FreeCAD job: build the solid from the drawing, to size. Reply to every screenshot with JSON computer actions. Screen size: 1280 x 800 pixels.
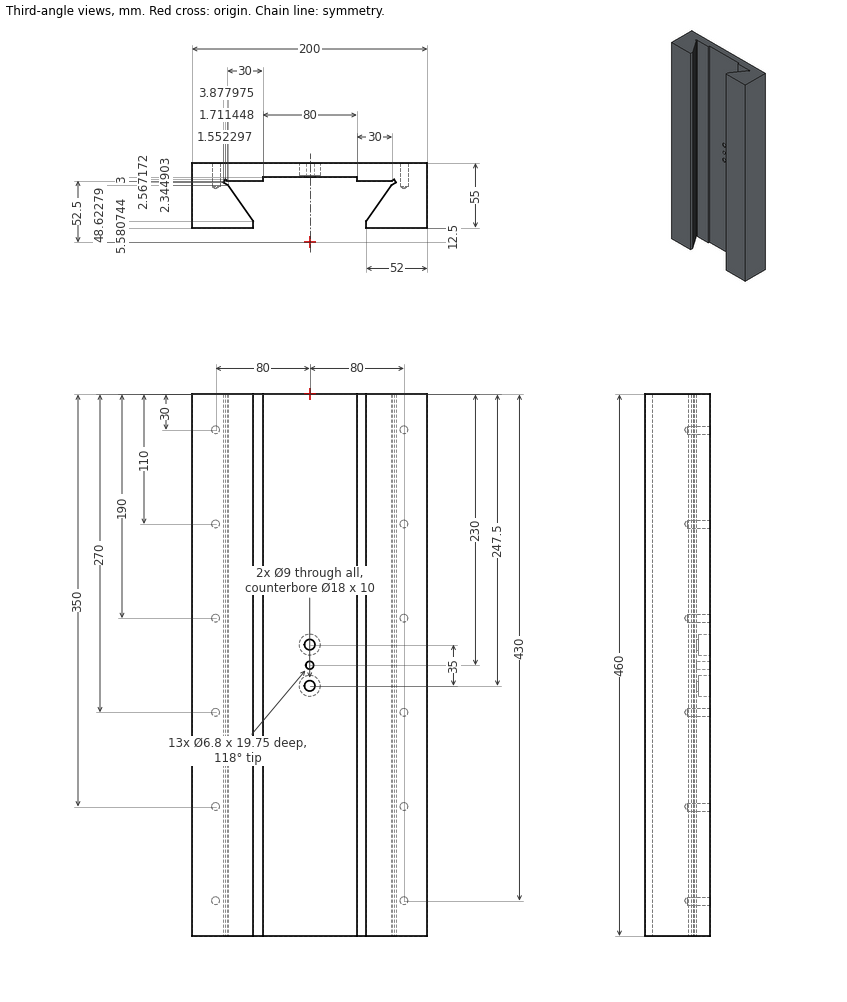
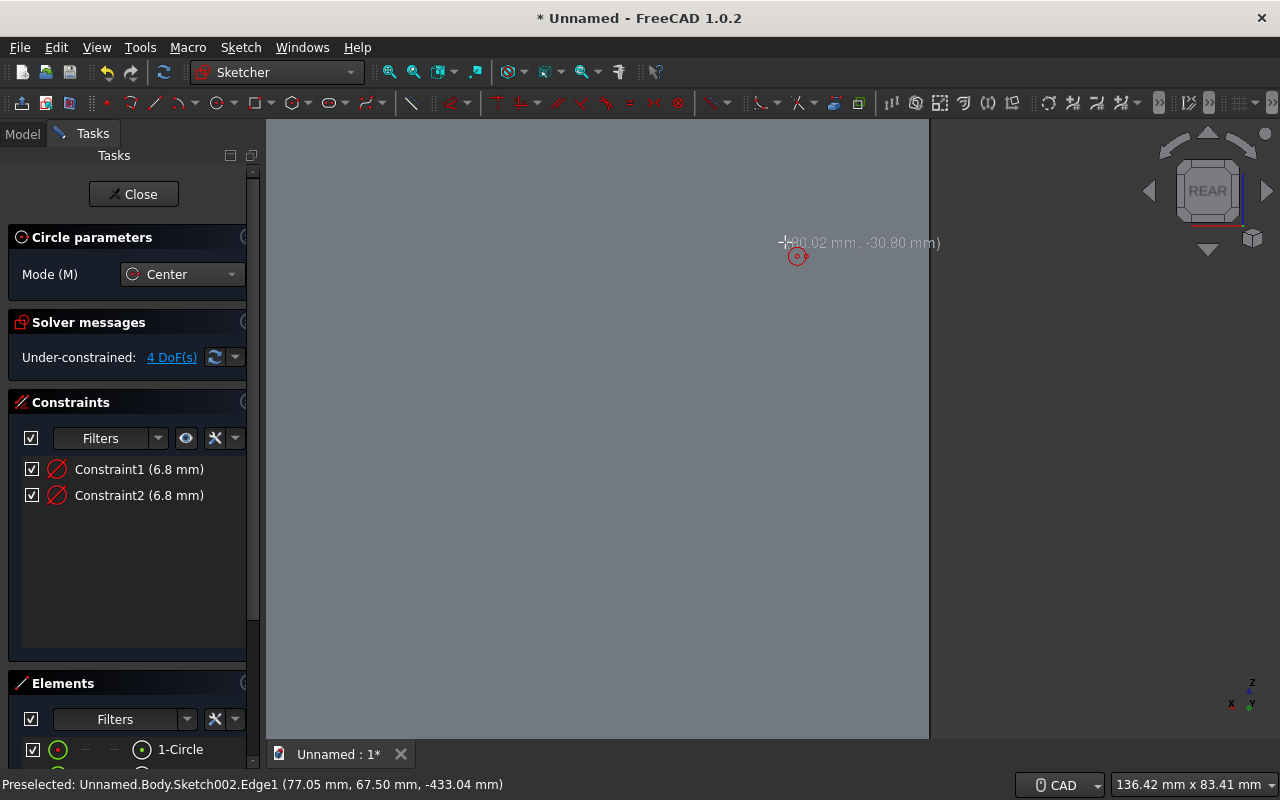
{"action": "scroll", "coordinate": [786, 241], "scroll_direction": "down", "scroll_amount": 10}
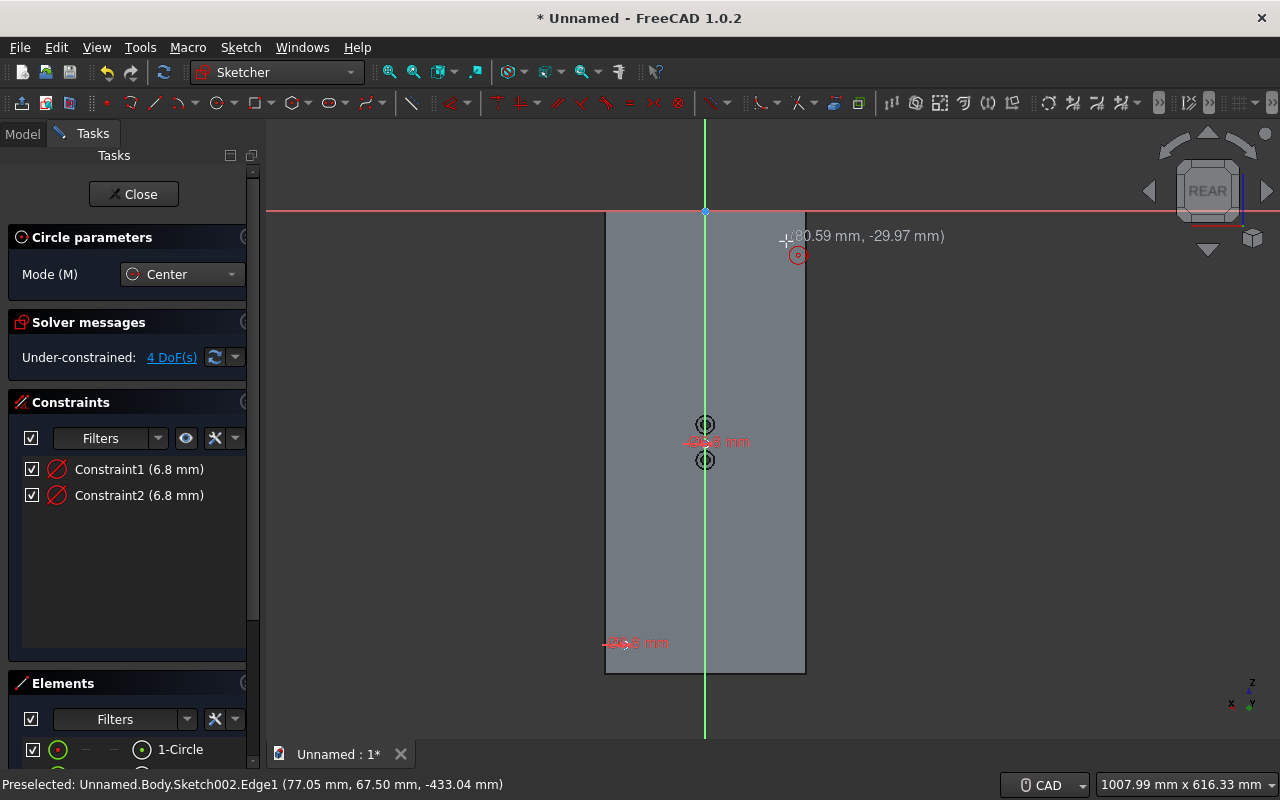
{"action": "left_click", "coordinate": [786, 241]}
{"action": "mouse_move", "coordinate": [788, 239]}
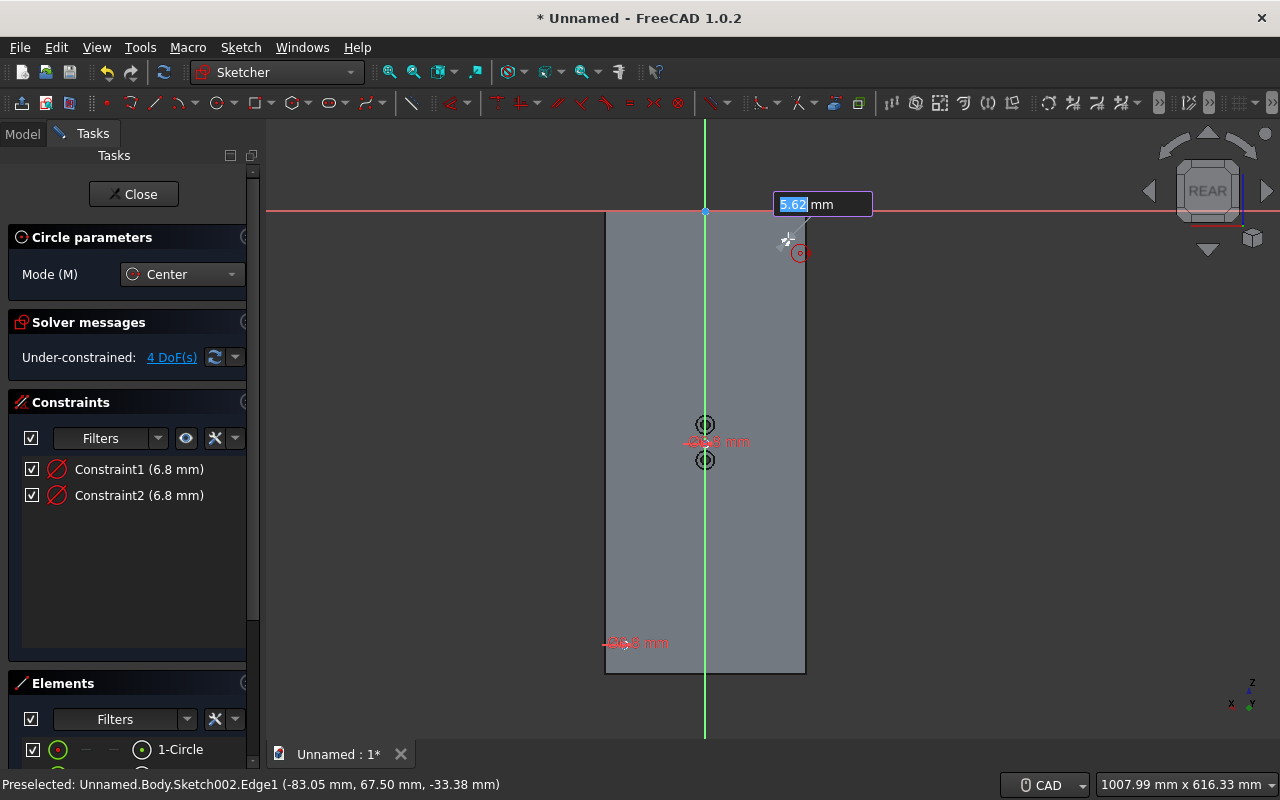
{"action": "type", "text": "6.8"}
{"action": "key", "text": "Return"}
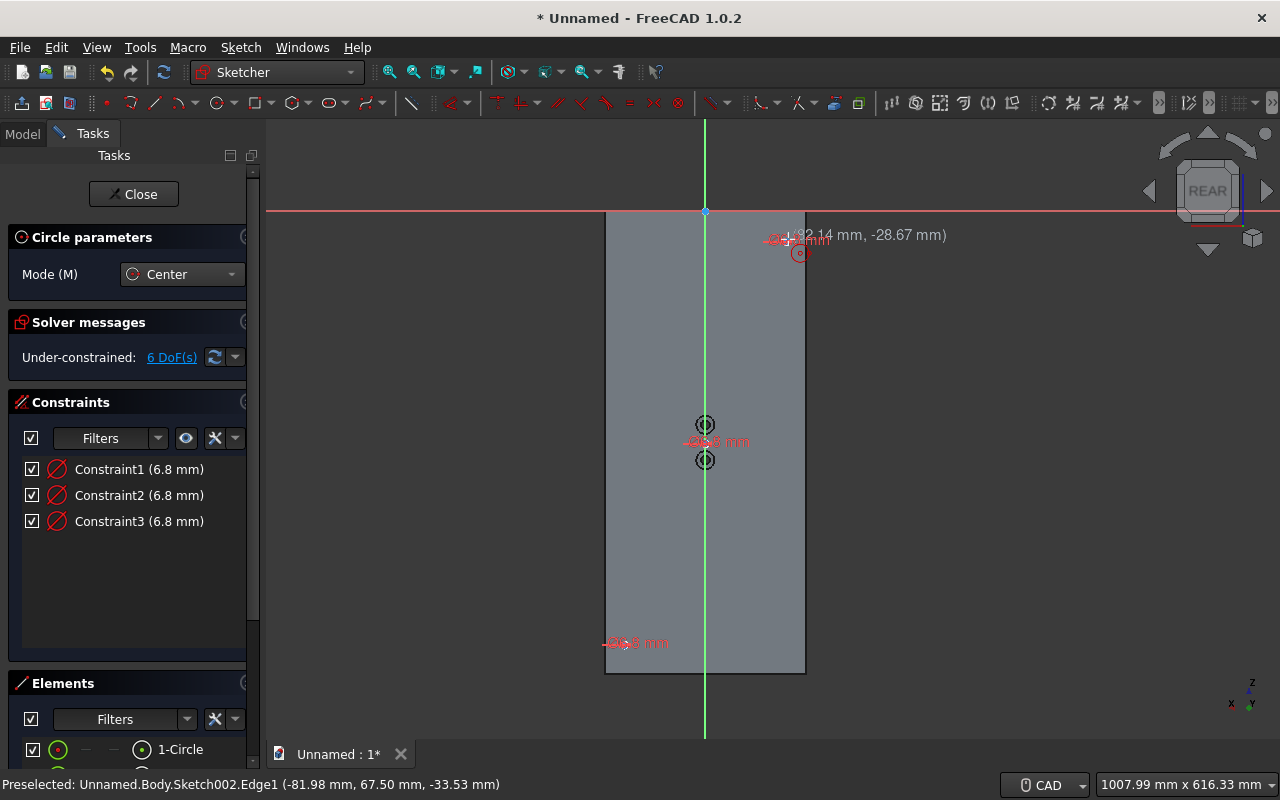
{"action": "scroll", "coordinate": [786, 644], "scroll_direction": "up", "scroll_amount": 10}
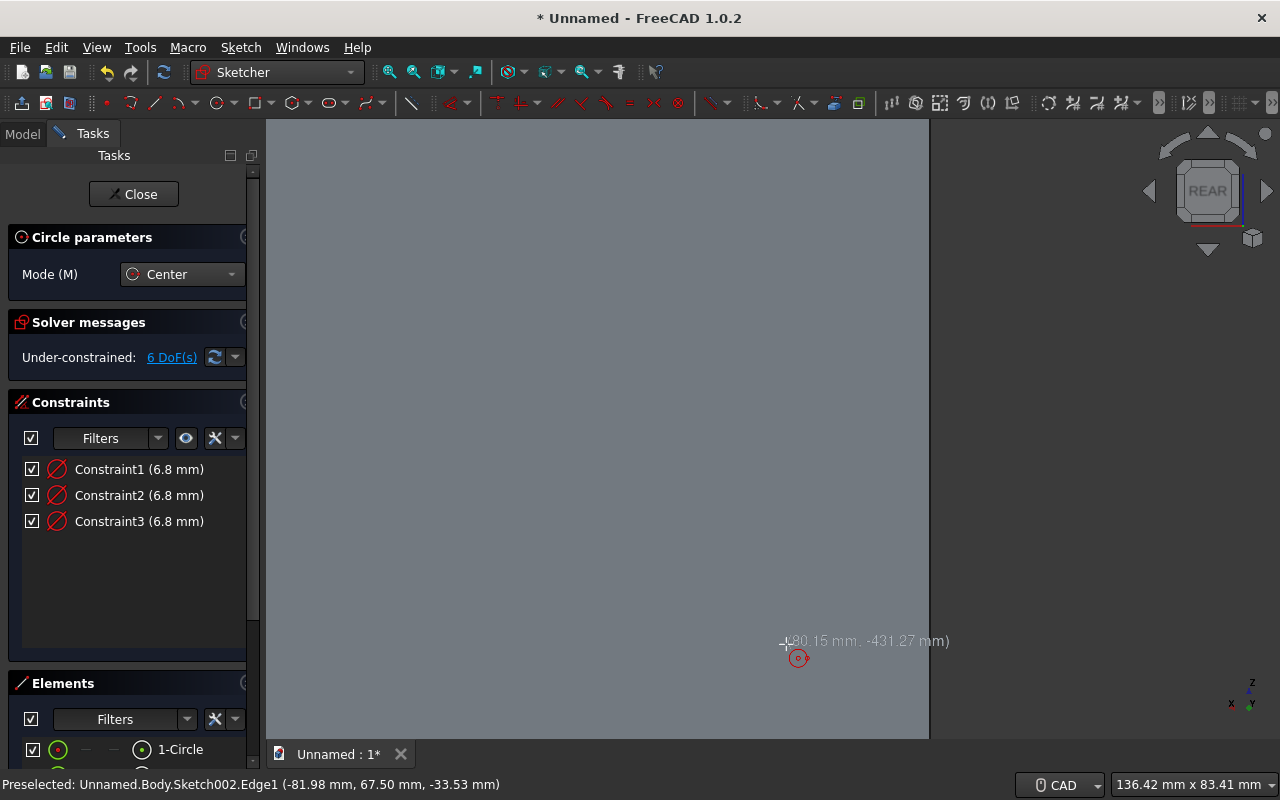
{"action": "scroll", "coordinate": [786, 645], "scroll_direction": "down", "scroll_amount": 10}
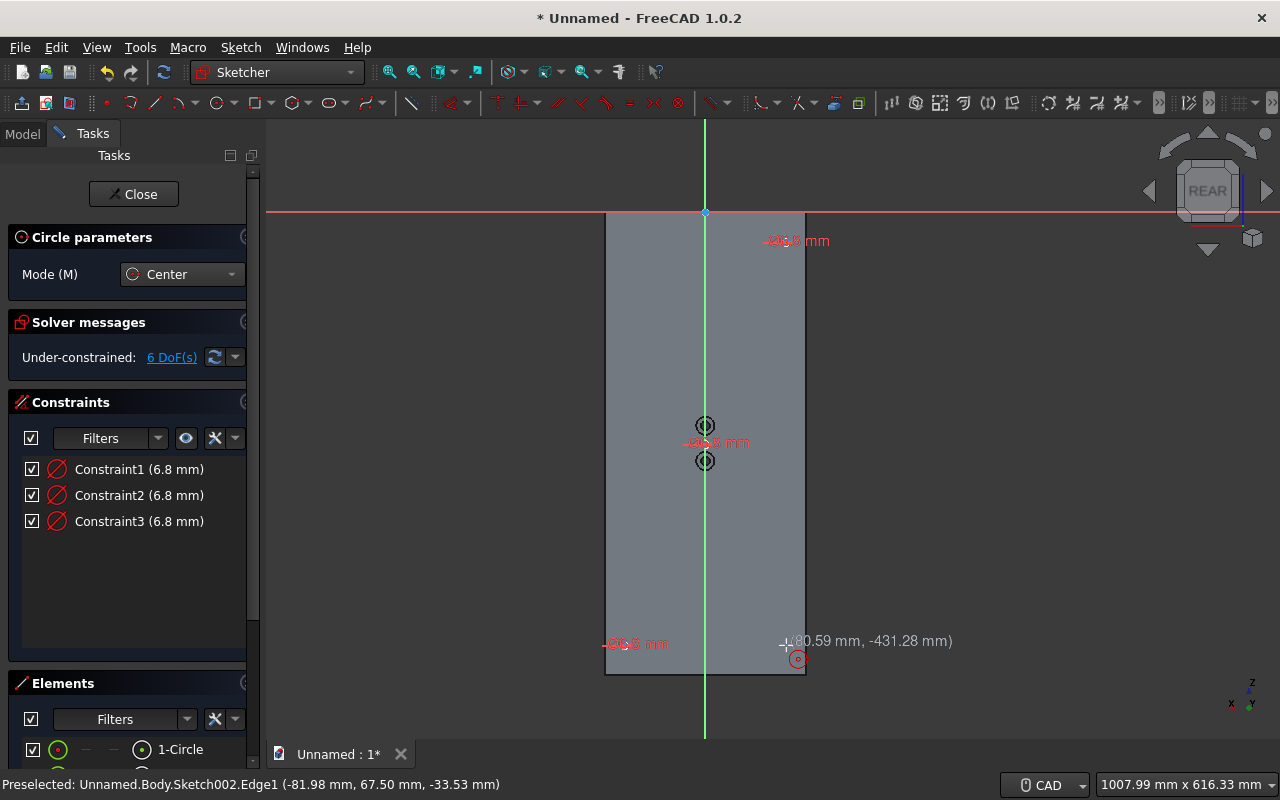
{"action": "left_click", "coordinate": [786, 645]}
{"action": "mouse_move", "coordinate": [788, 642]}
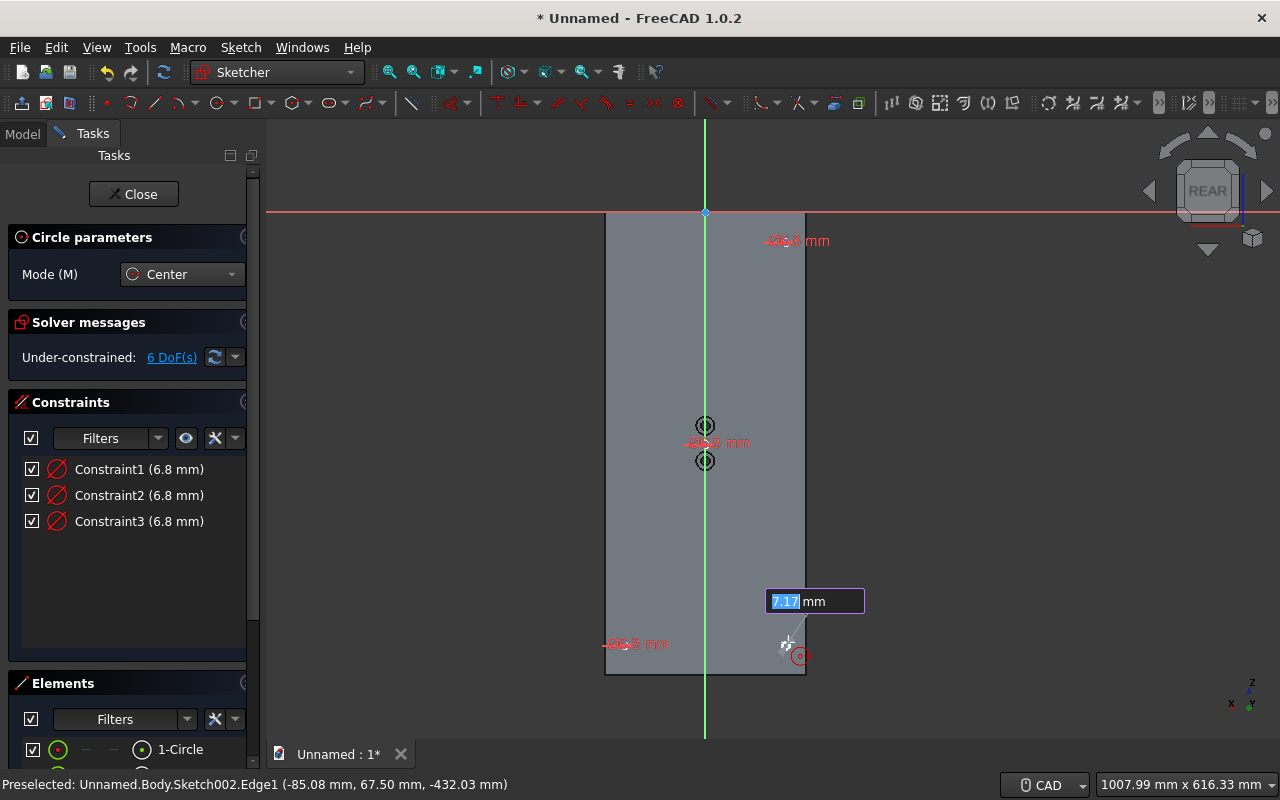
{"action": "type", "text": "6.8"}
{"action": "key", "text": "Return"}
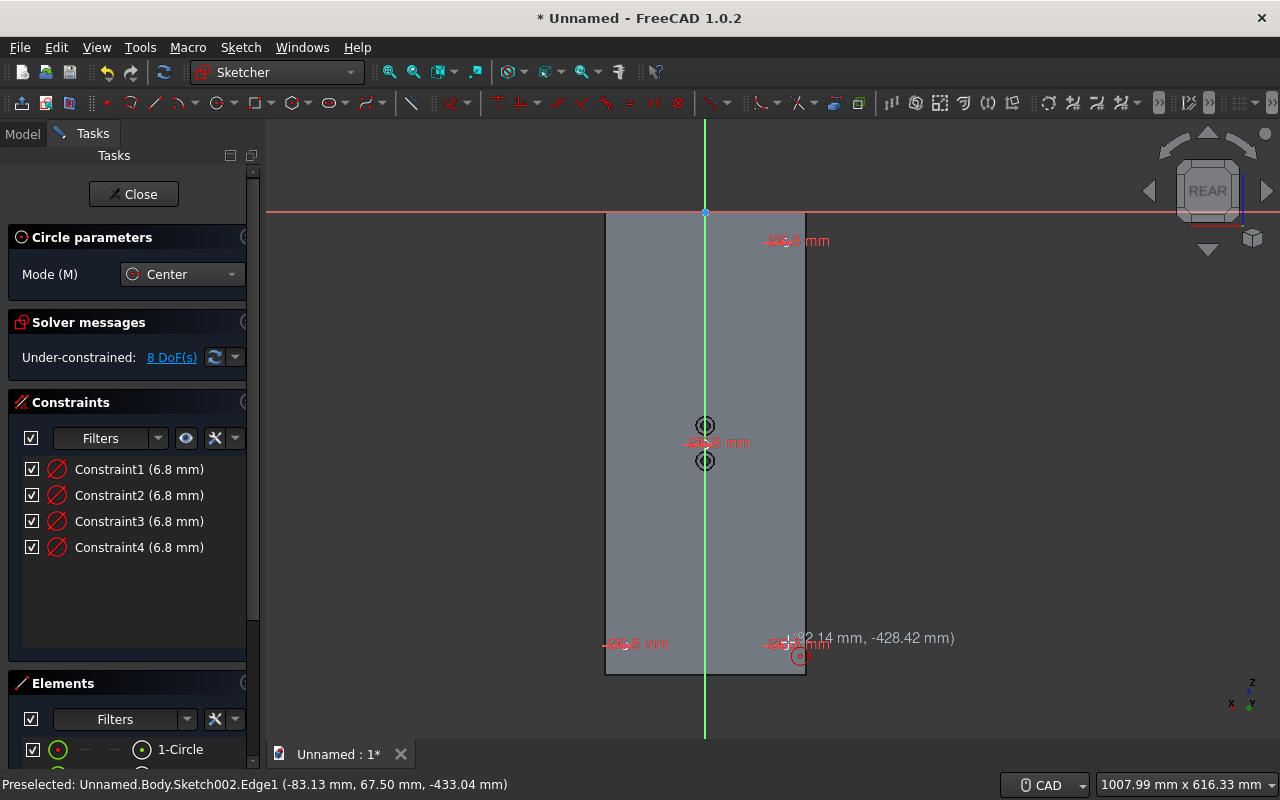
{"action": "scroll", "coordinate": [625, 242], "scroll_direction": "up", "scroll_amount": 10}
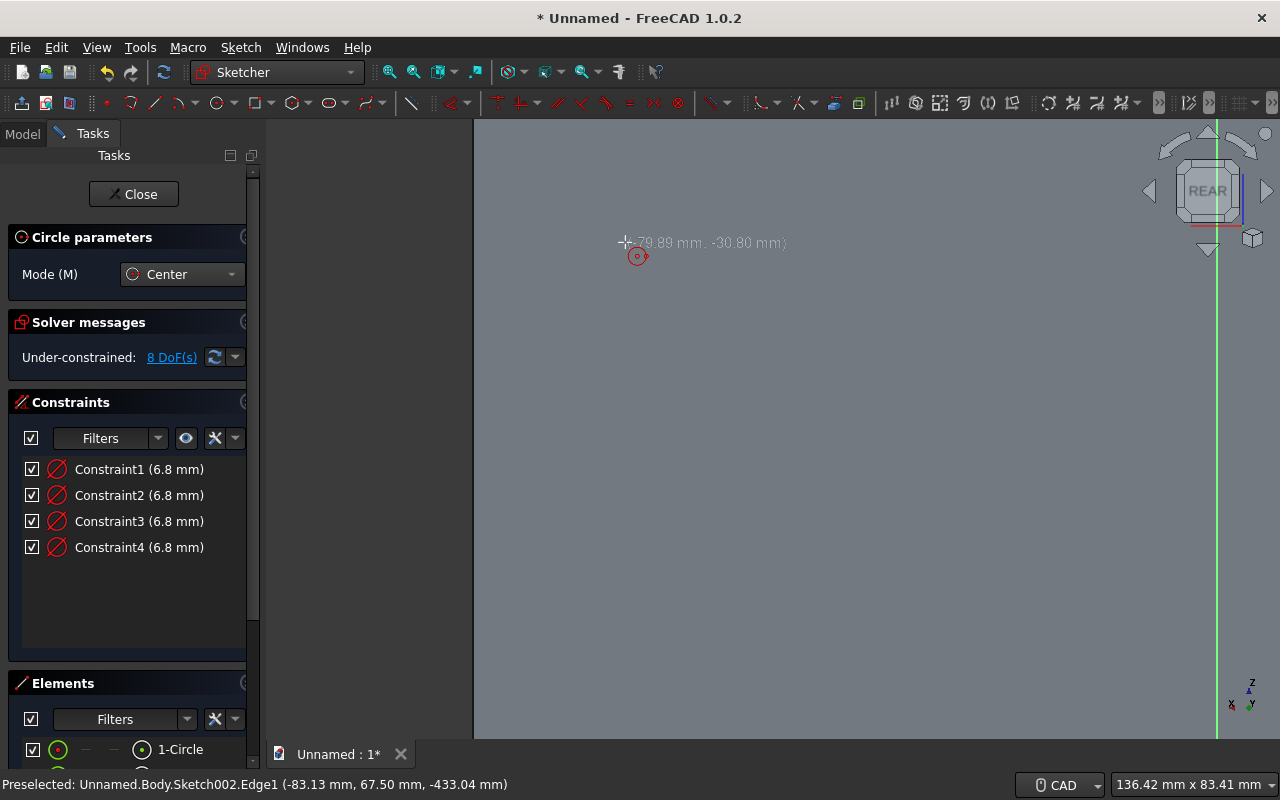
{"action": "scroll", "coordinate": [624, 241], "scroll_direction": "down", "scroll_amount": 10}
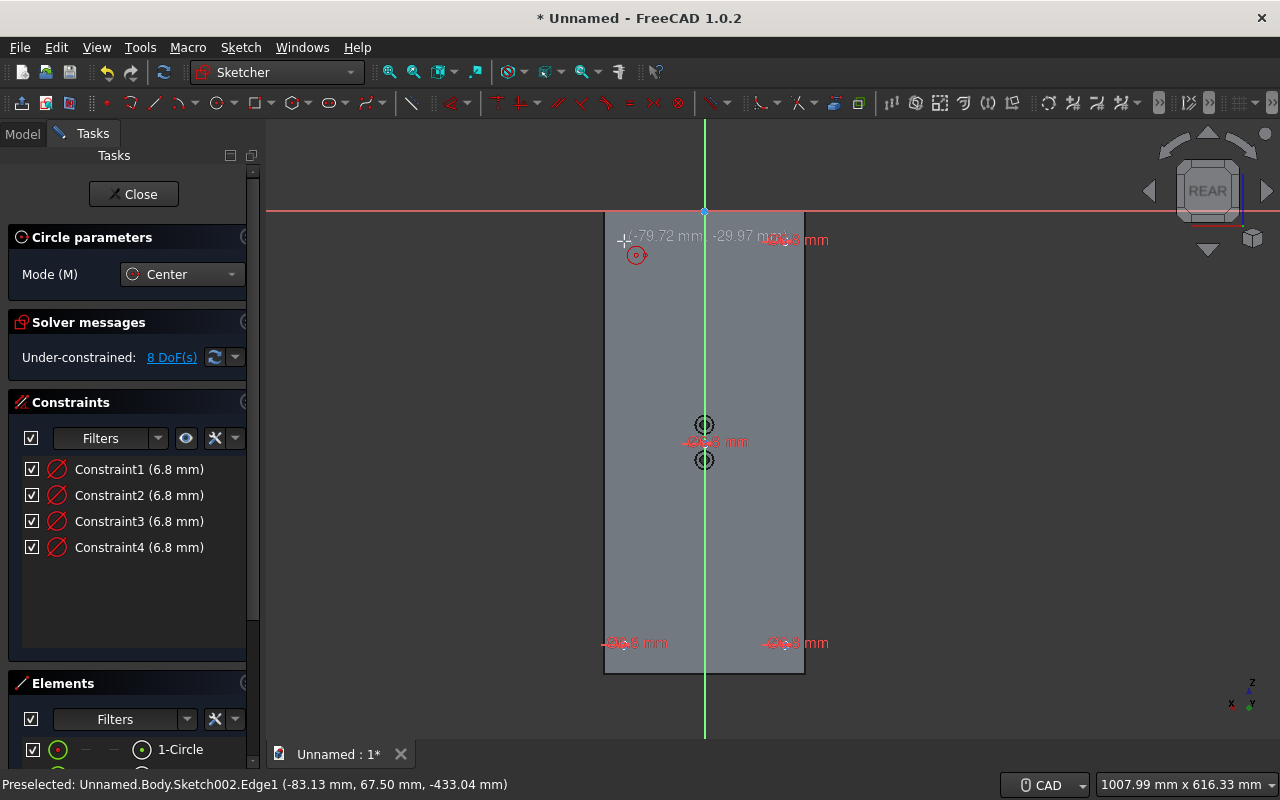
{"action": "left_click", "coordinate": [624, 241]}
{"action": "mouse_move", "coordinate": [626, 239]}